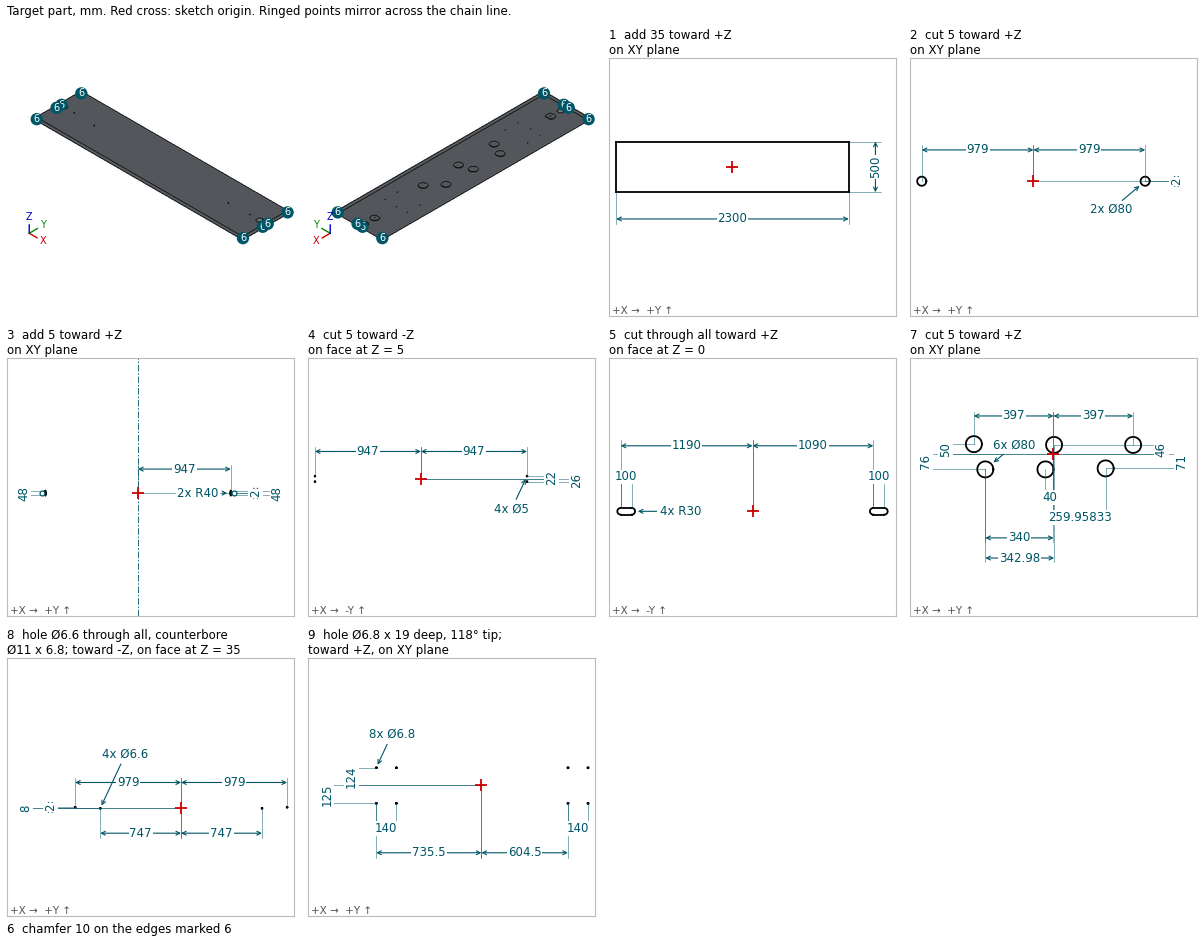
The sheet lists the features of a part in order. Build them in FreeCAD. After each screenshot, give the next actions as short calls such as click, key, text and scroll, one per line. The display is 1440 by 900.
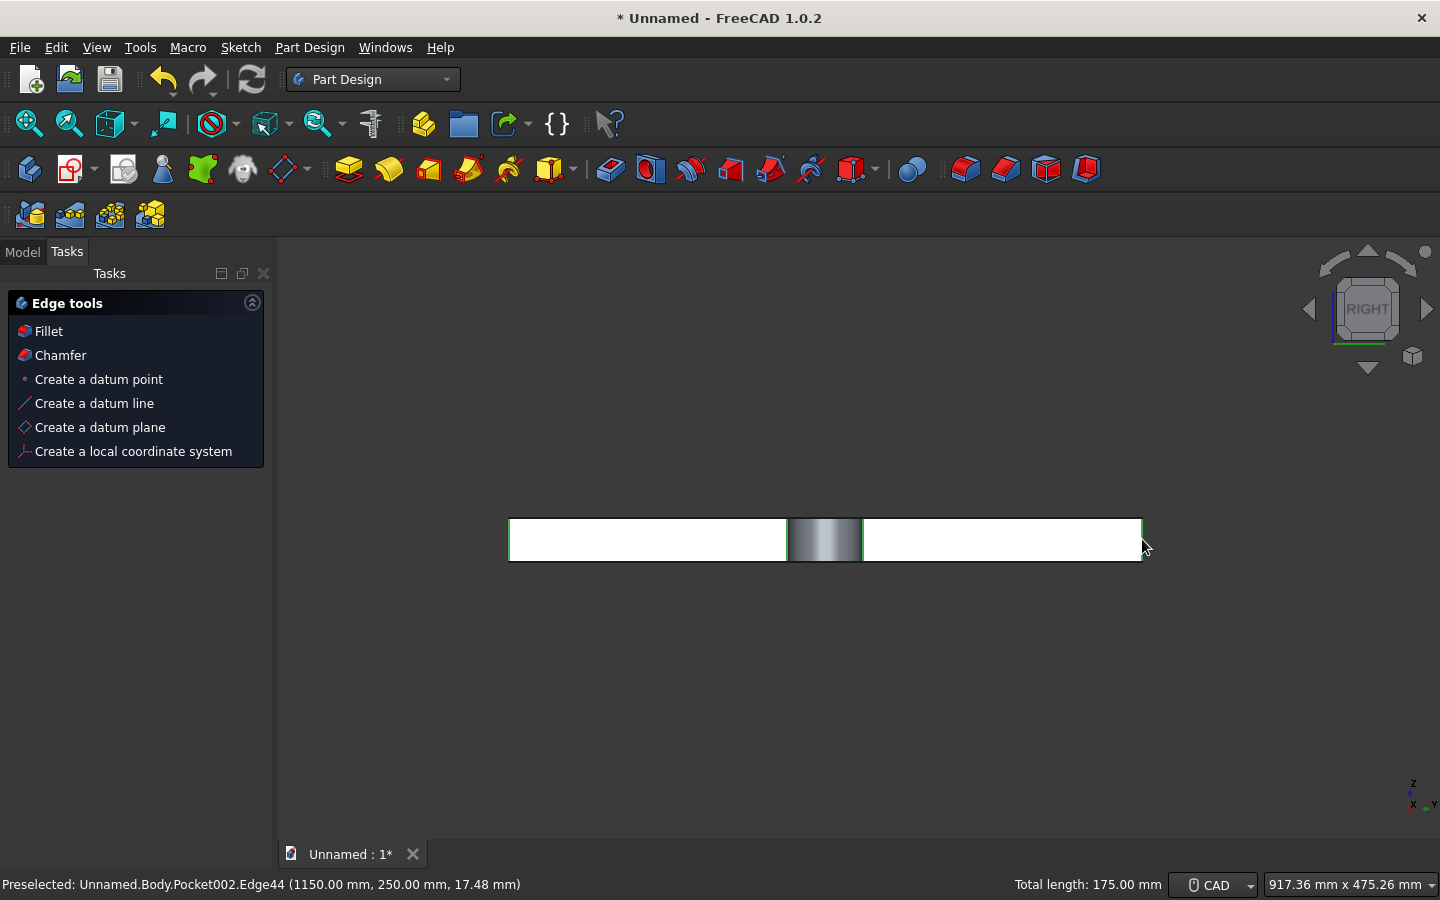
click(30, 124)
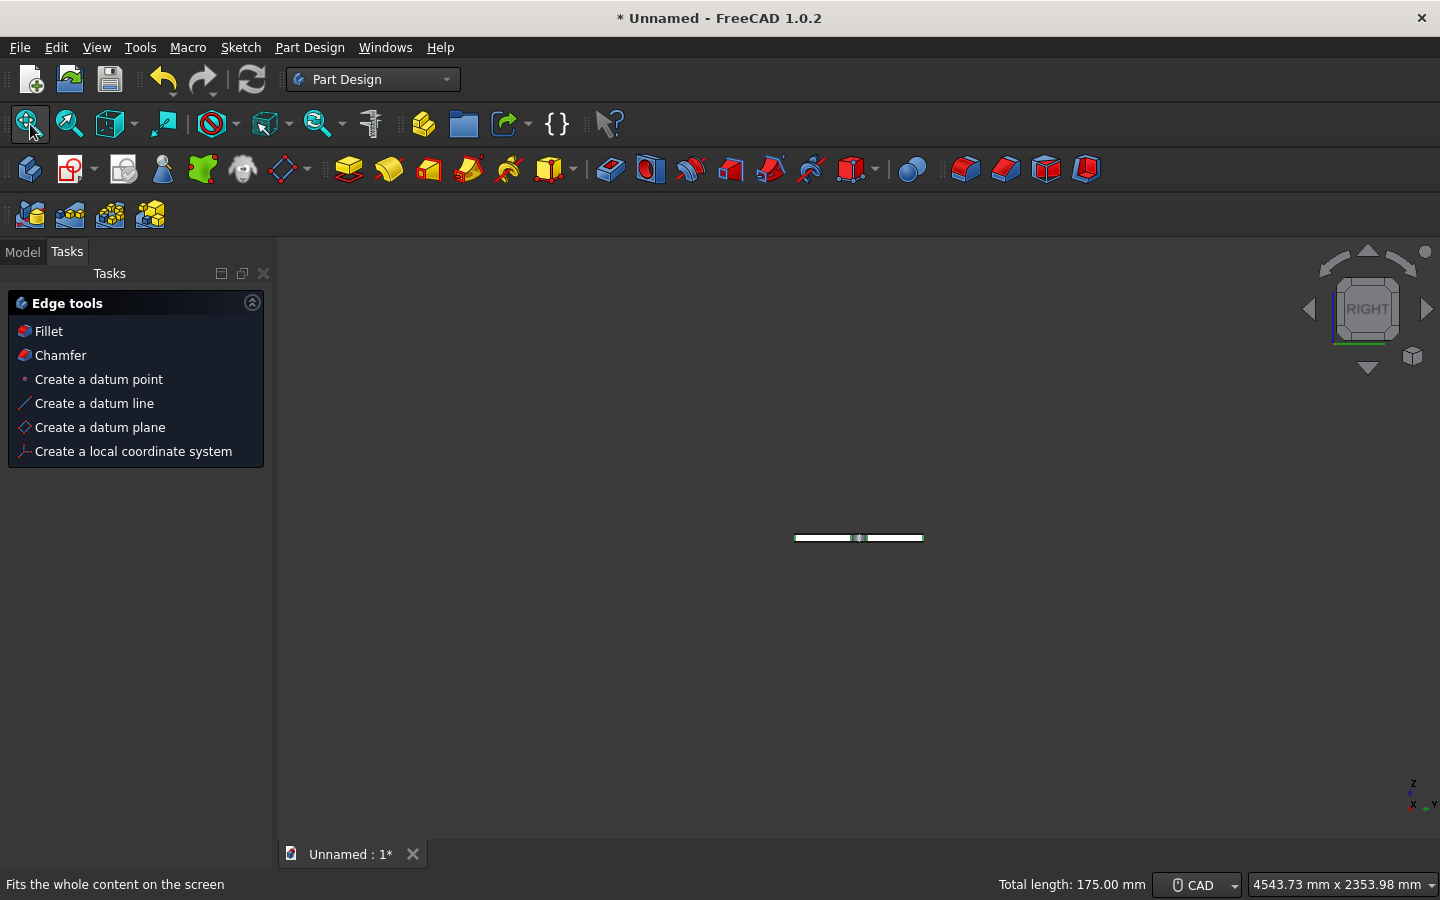
key(5)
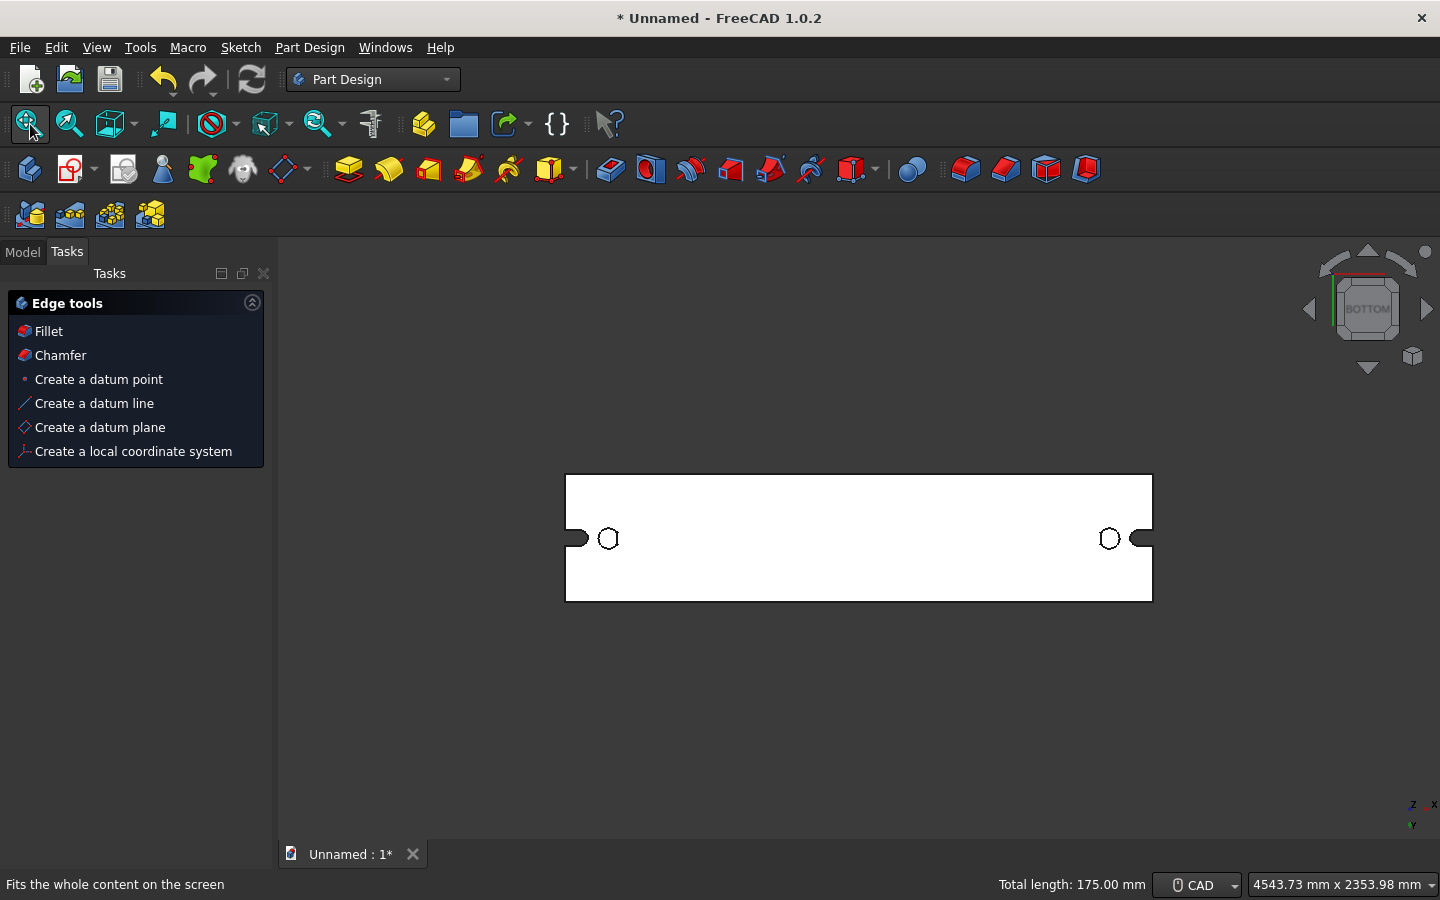
scroll(565, 545, up, 8)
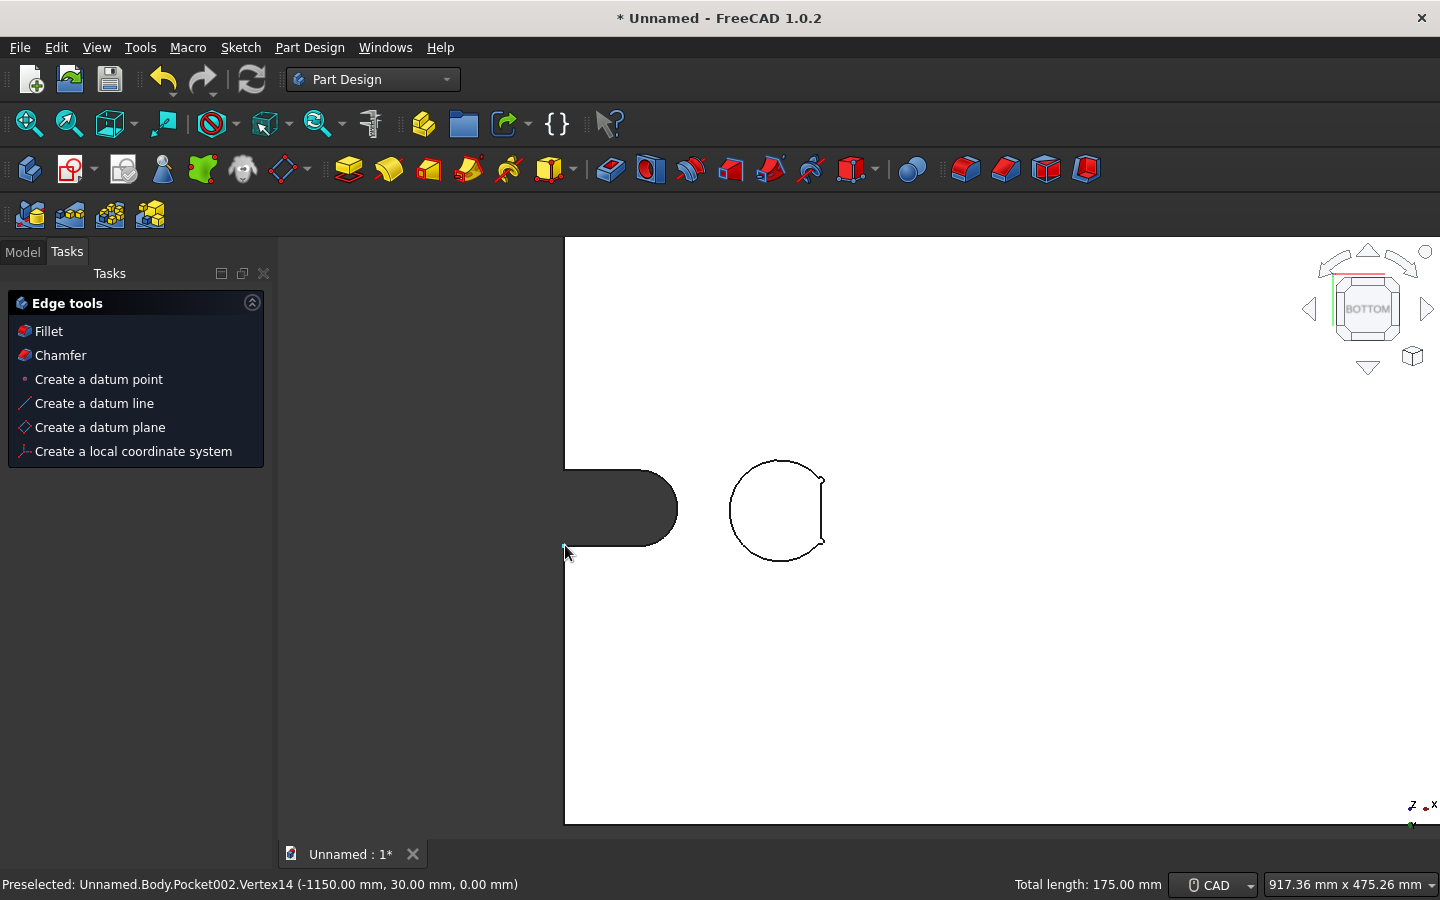
key(v)
key(f)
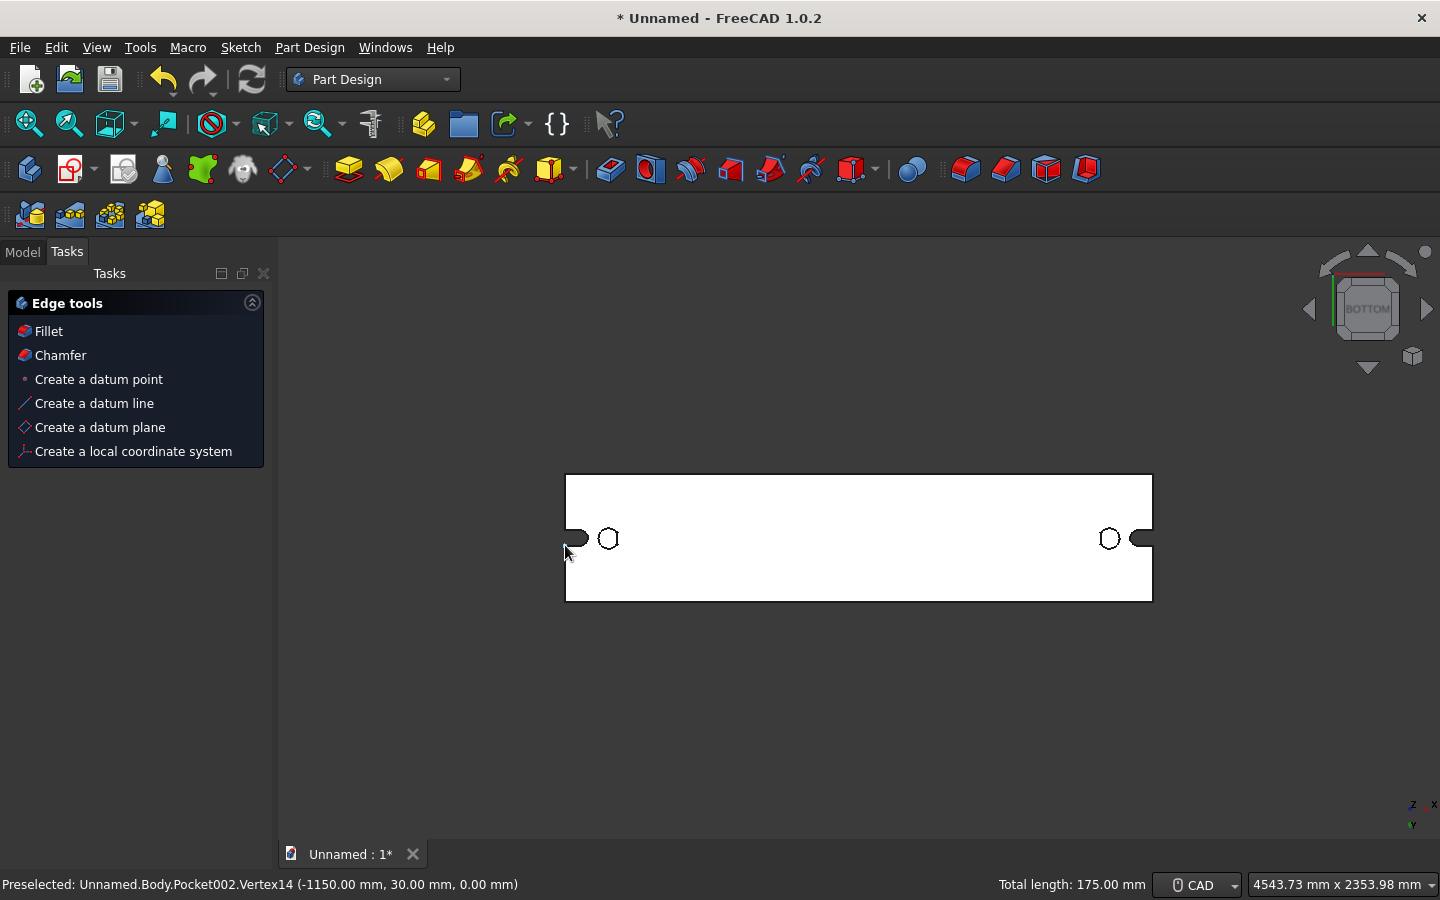
key(4)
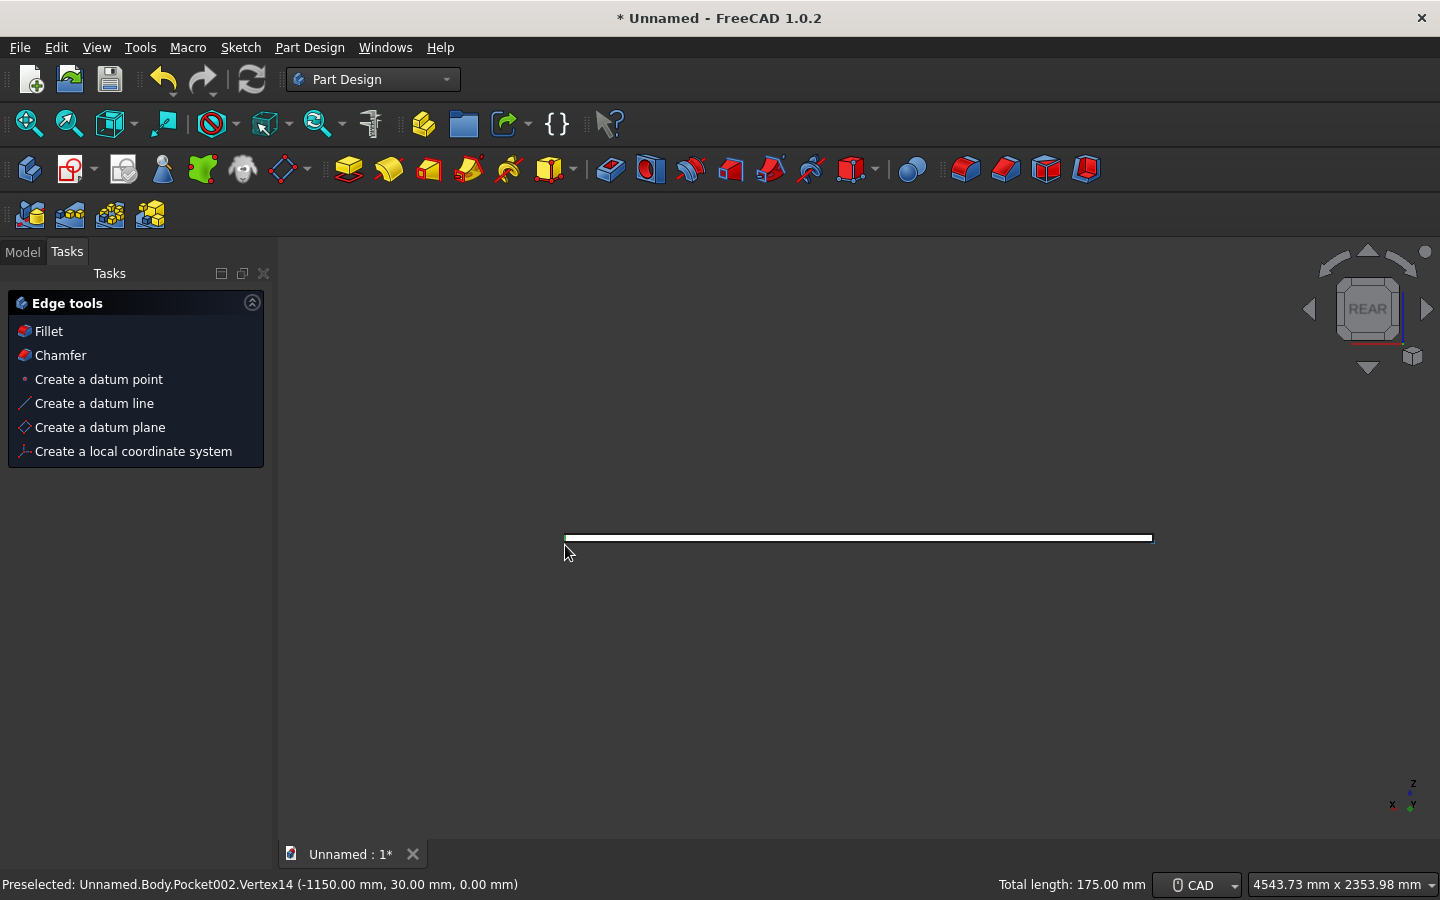
scroll(1153, 537, up, 8)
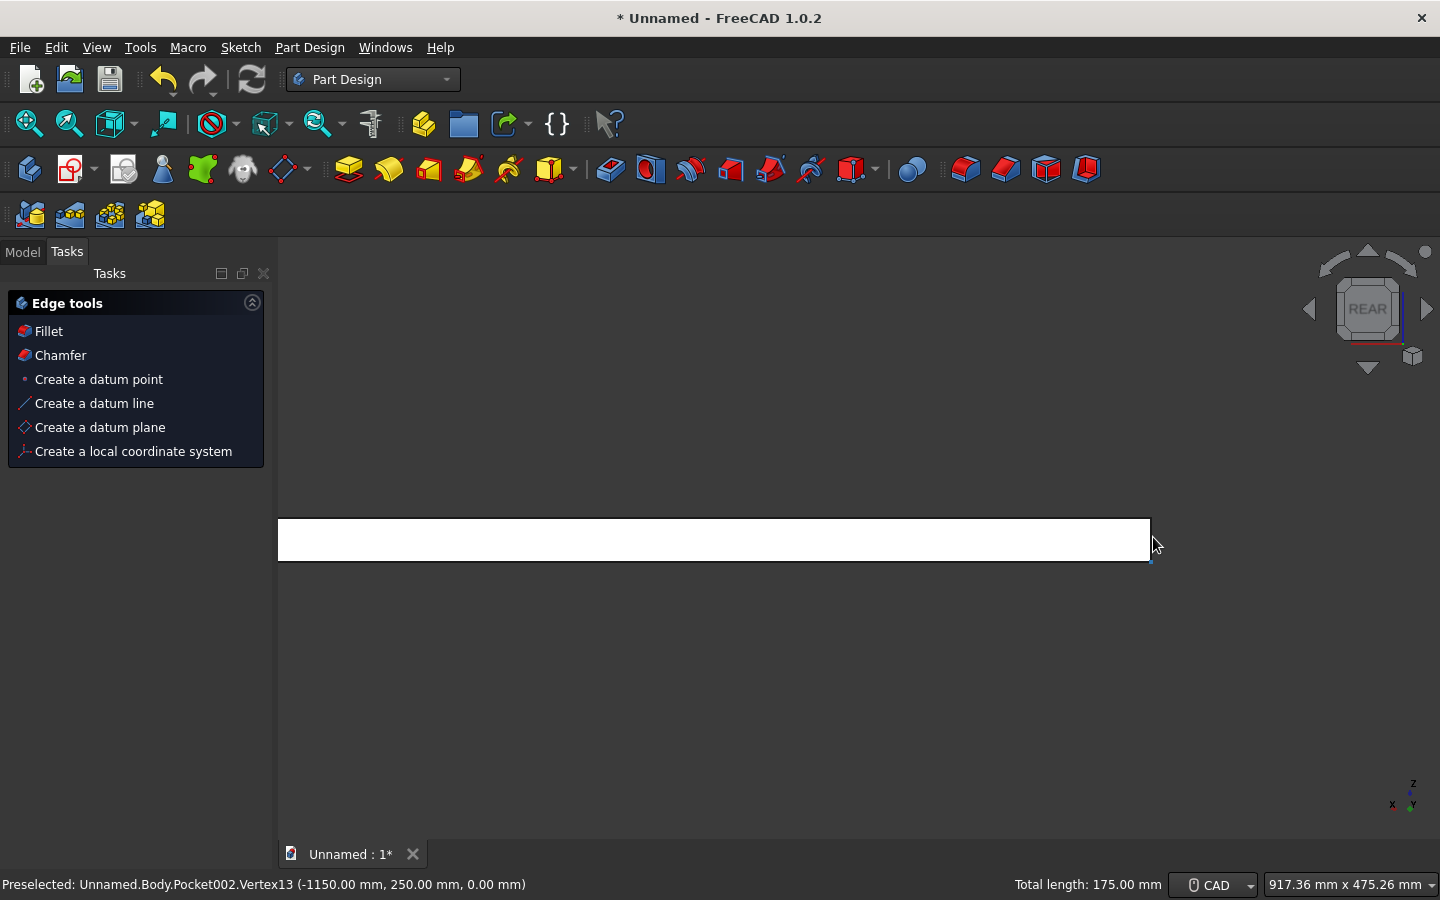
click(1151, 539, ctrl)